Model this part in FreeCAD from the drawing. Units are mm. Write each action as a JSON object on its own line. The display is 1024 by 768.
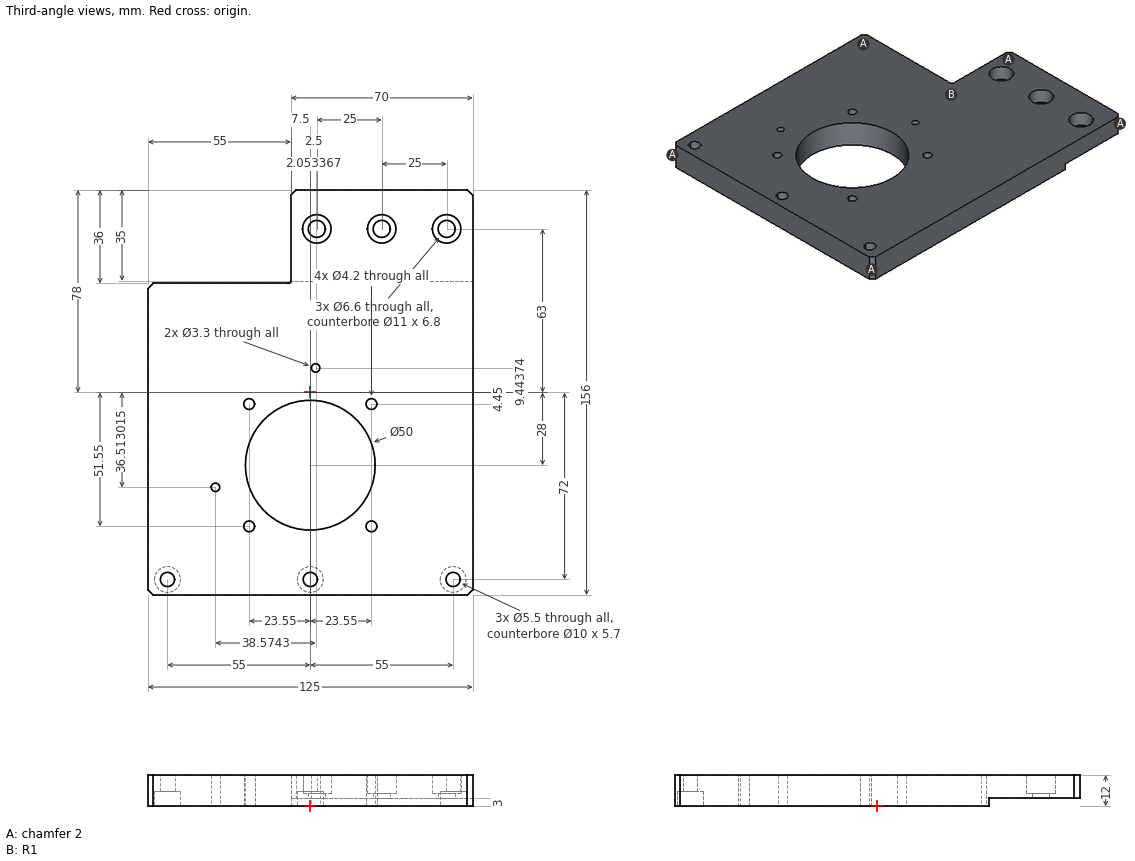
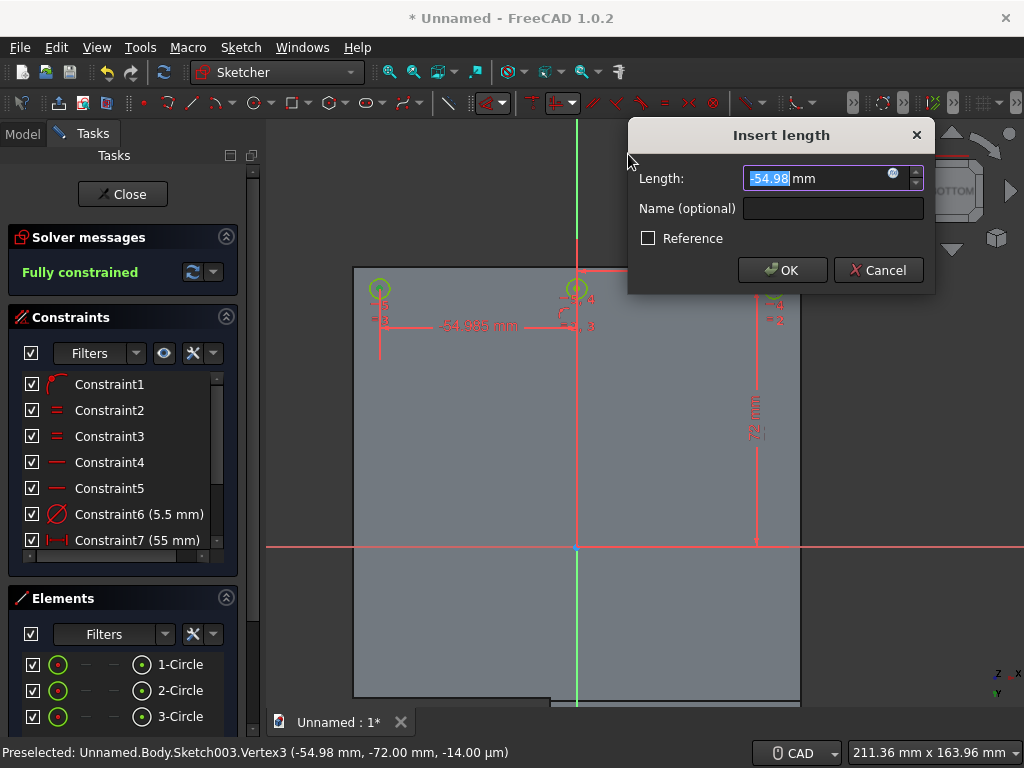
{"action": "type", "text": "-55"}
{"action": "key", "text": "Return"}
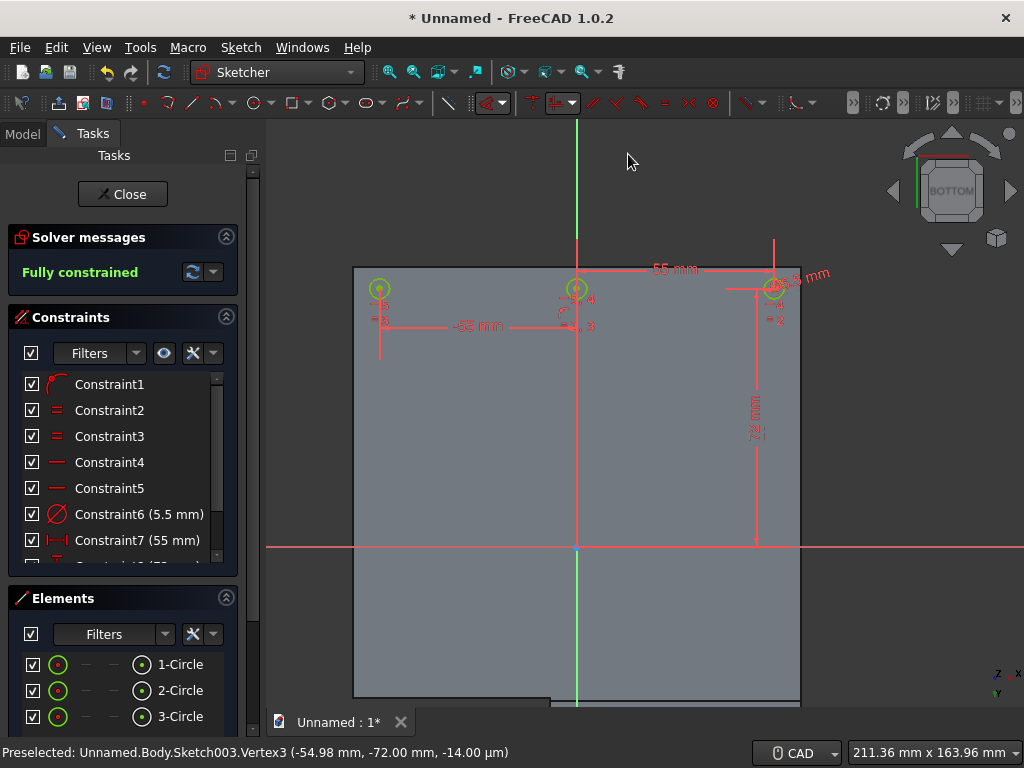
{"action": "left_click", "coordinate": [123, 194]}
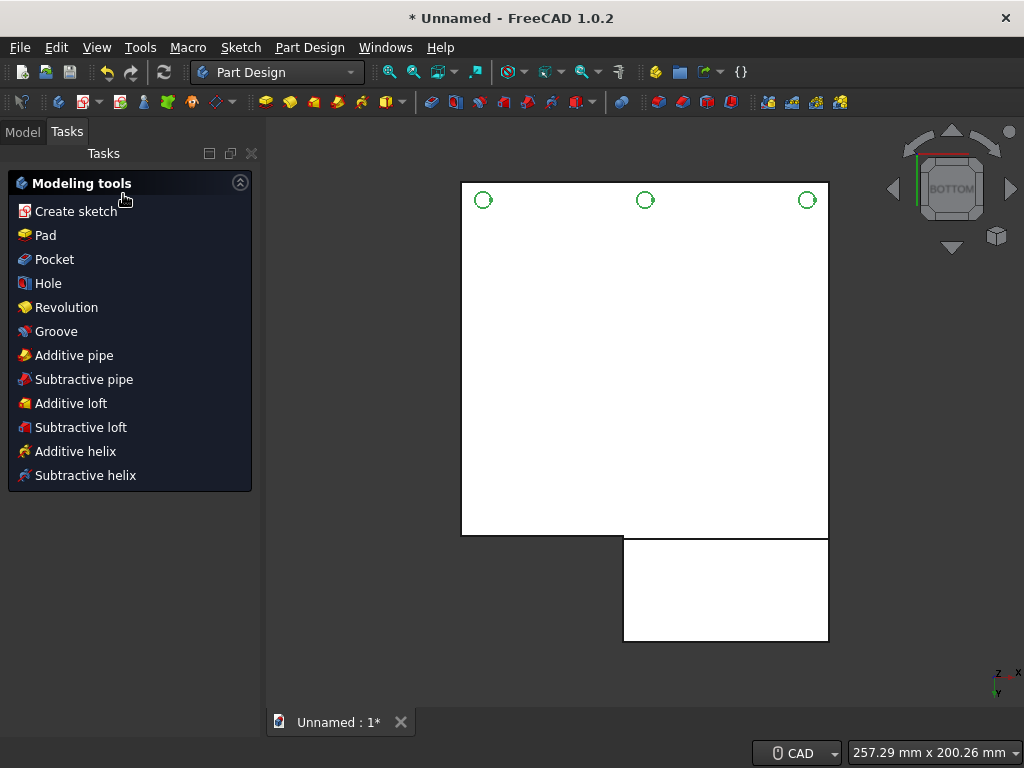
{"action": "left_click", "coordinate": [456, 102]}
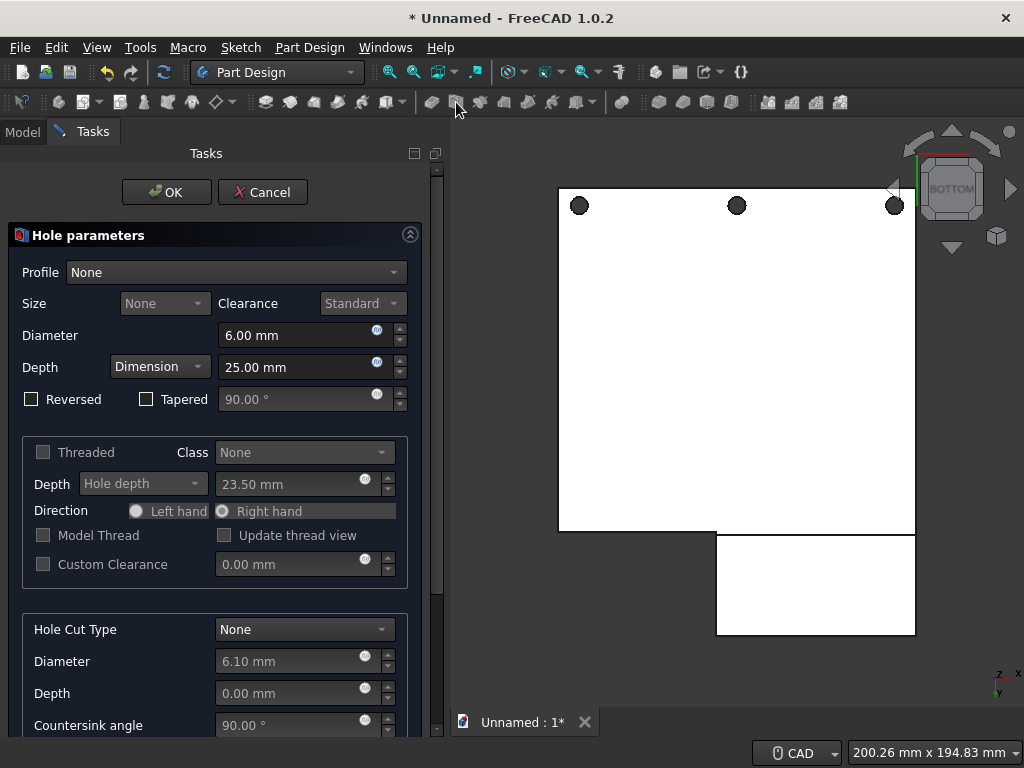
{"action": "triple_click", "coordinate": [305, 335]}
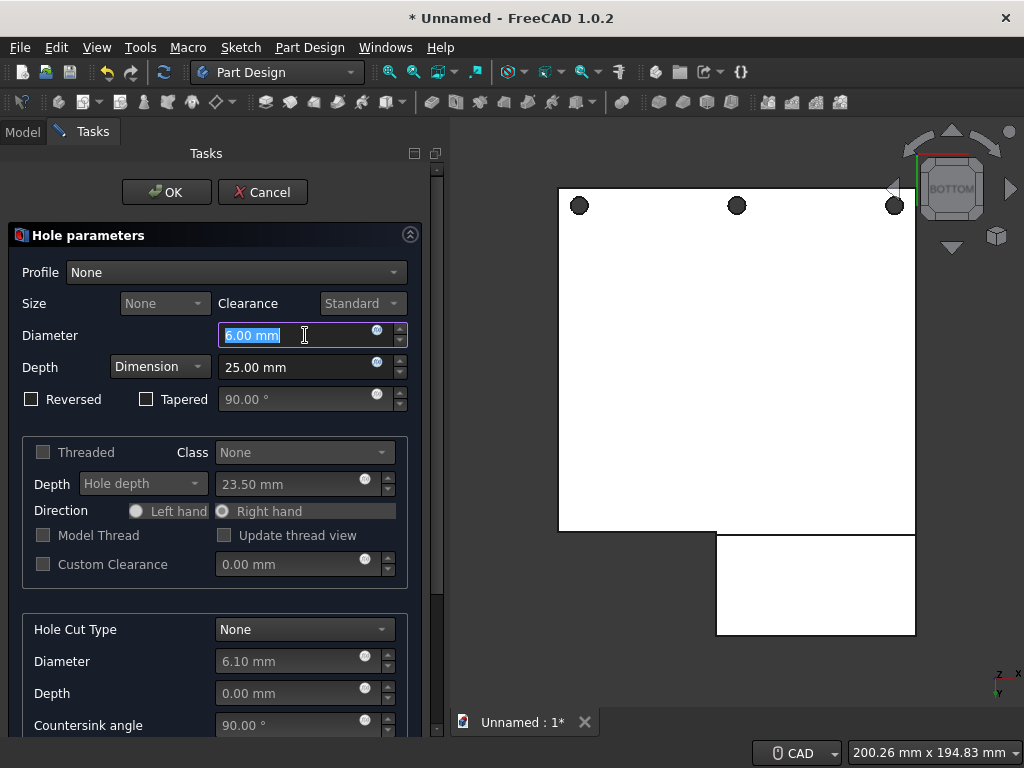
{"action": "type", "text": "5.5"}
{"action": "key", "text": "Tab"}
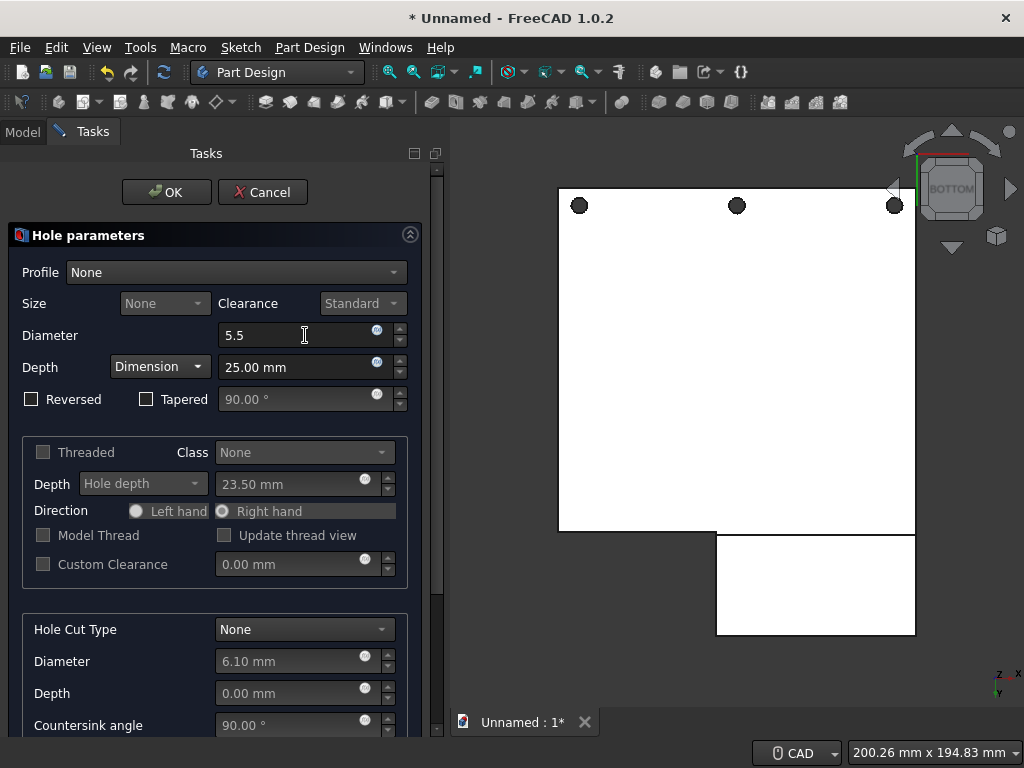
{"action": "left_click", "coordinate": [161, 366]}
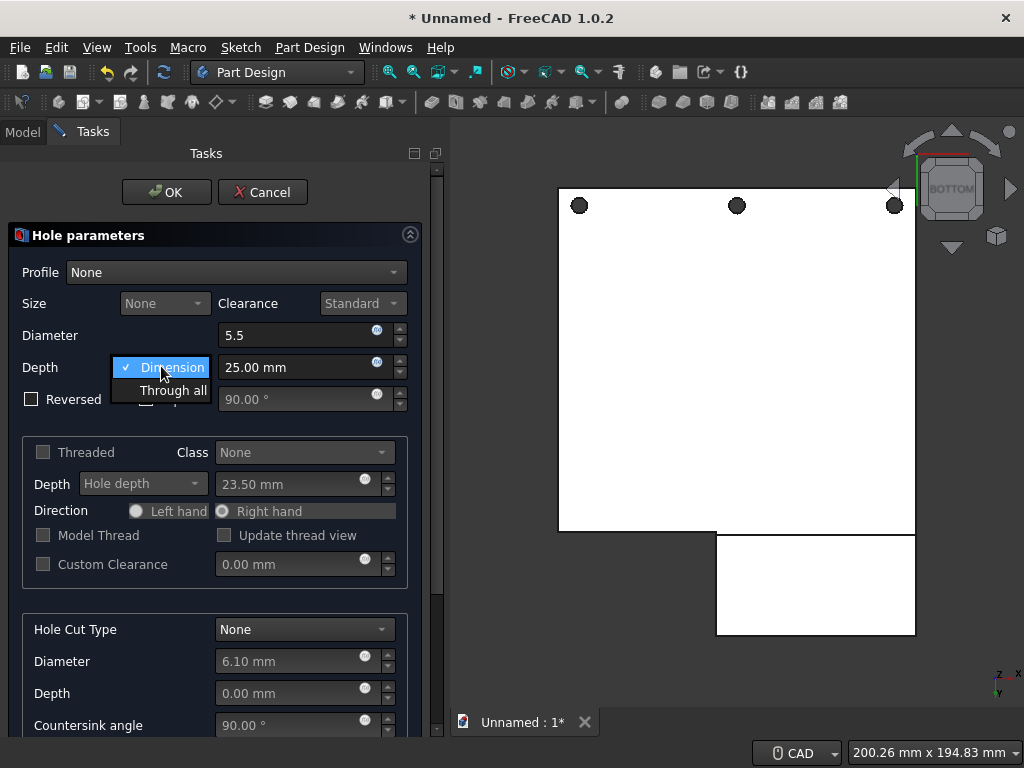
{"action": "left_click", "coordinate": [160, 390]}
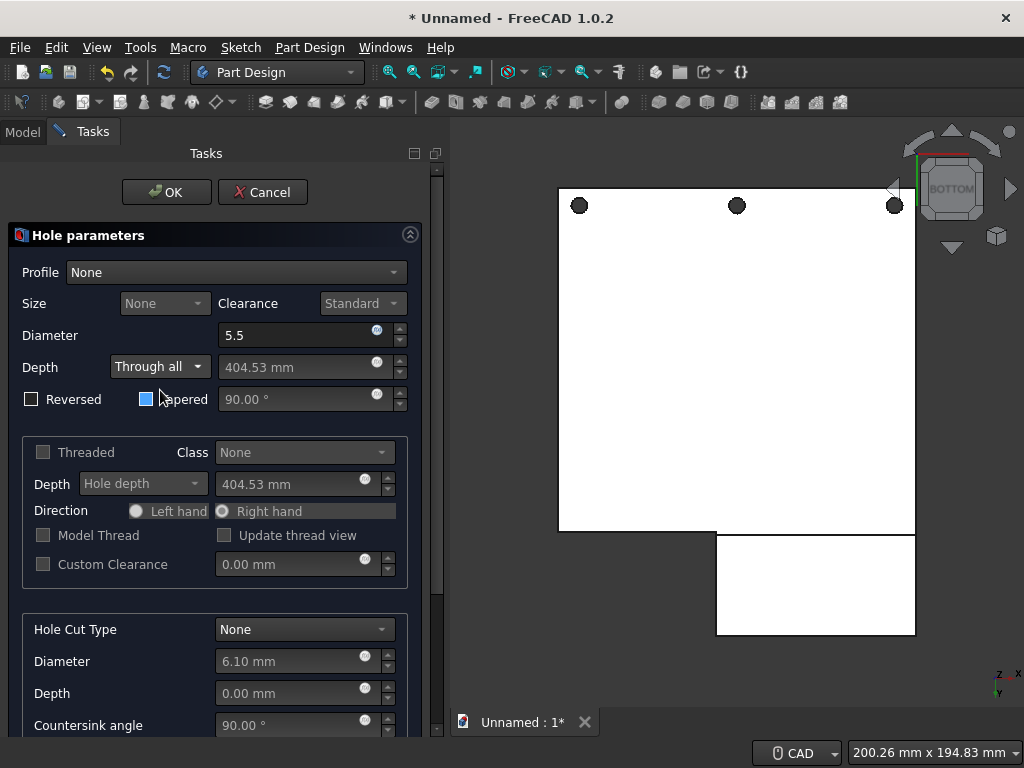
{"action": "left_click", "coordinate": [306, 630]}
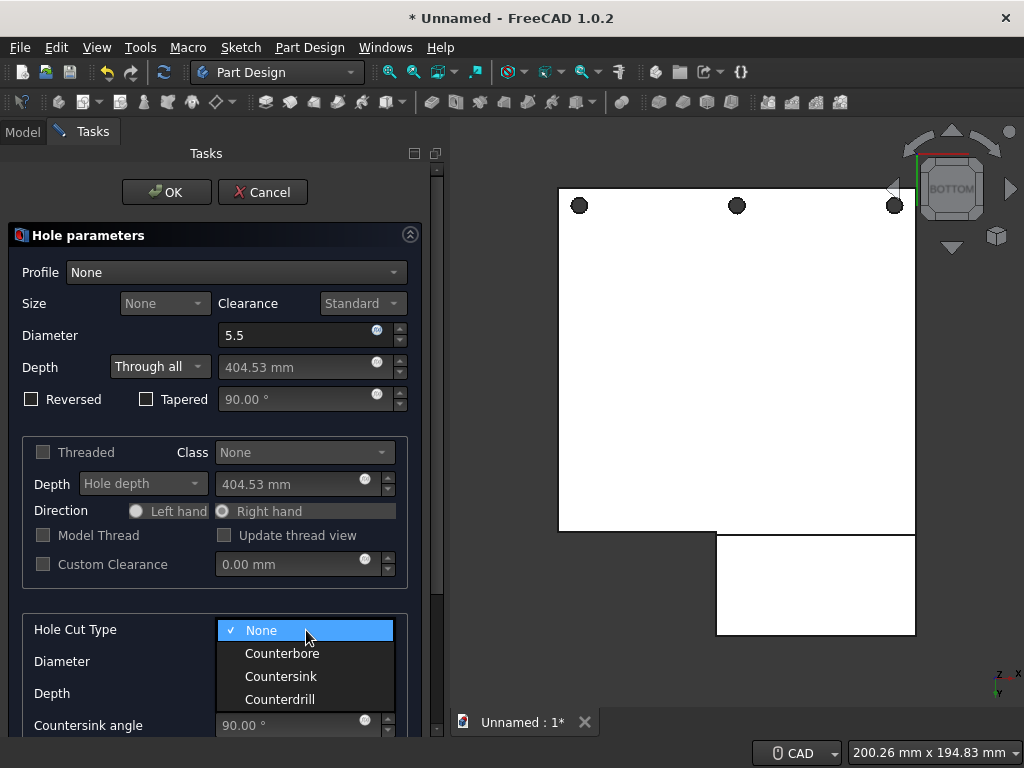
{"action": "left_click", "coordinate": [304, 654]}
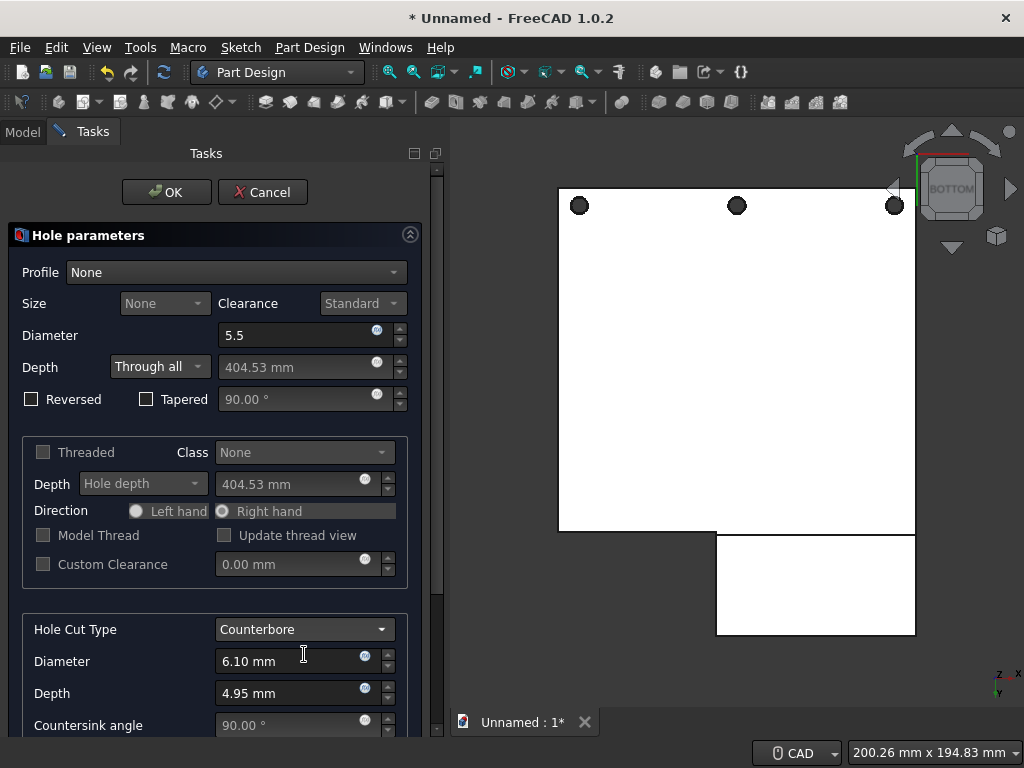
{"action": "triple_click", "coordinate": [298, 661]}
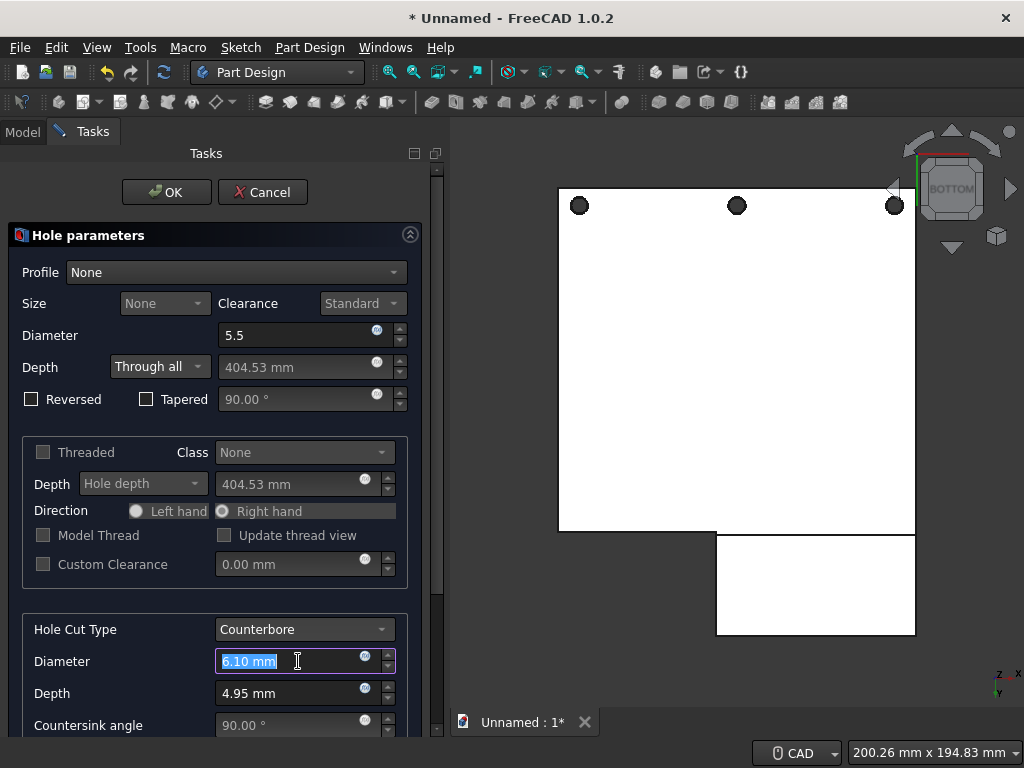
{"action": "type", "text": "10"}
{"action": "key", "text": "Tab"}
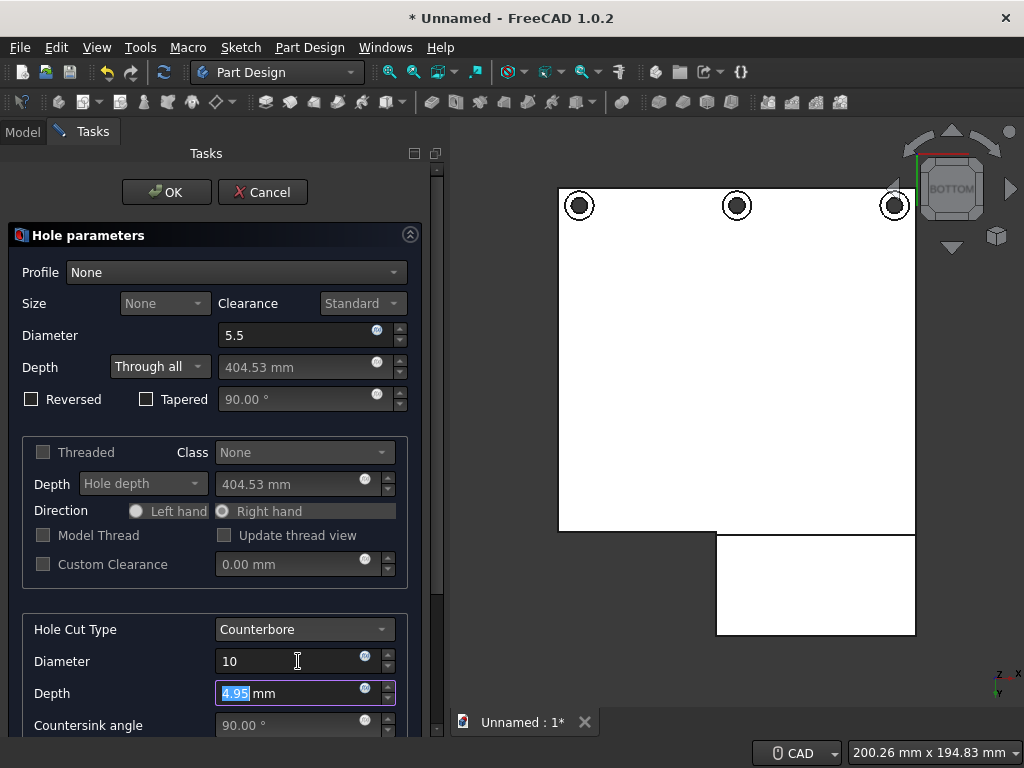
{"action": "type", "text": "5.7"}
{"action": "key", "text": "Tab"}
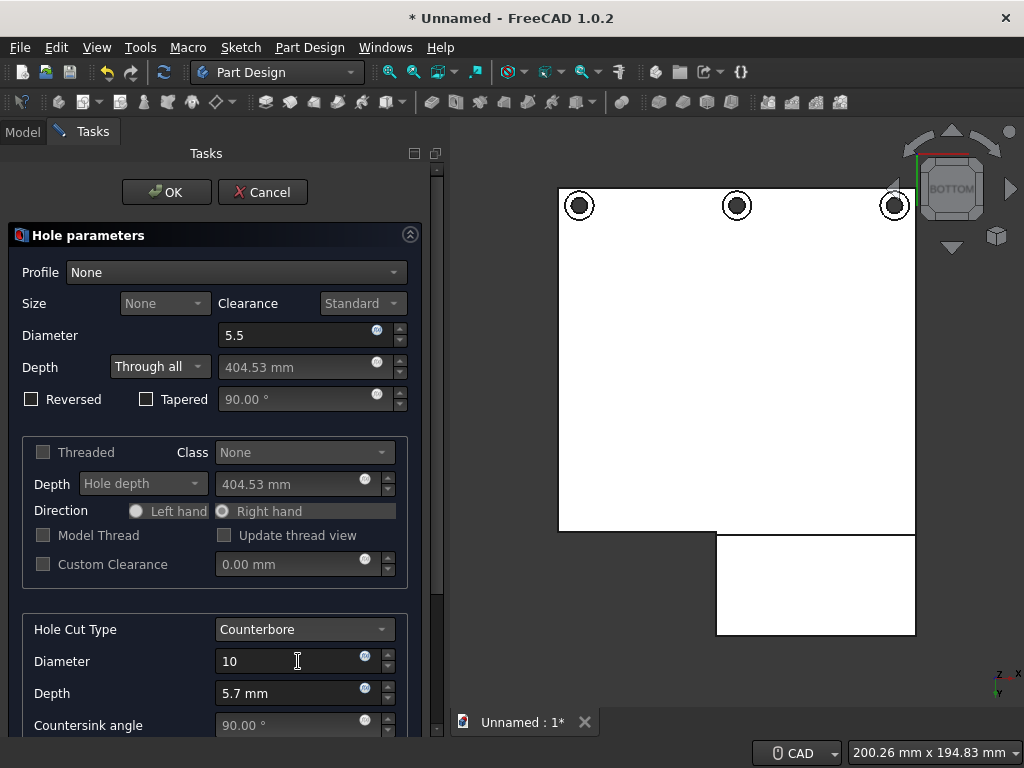
{"action": "left_click", "coordinate": [167, 192]}